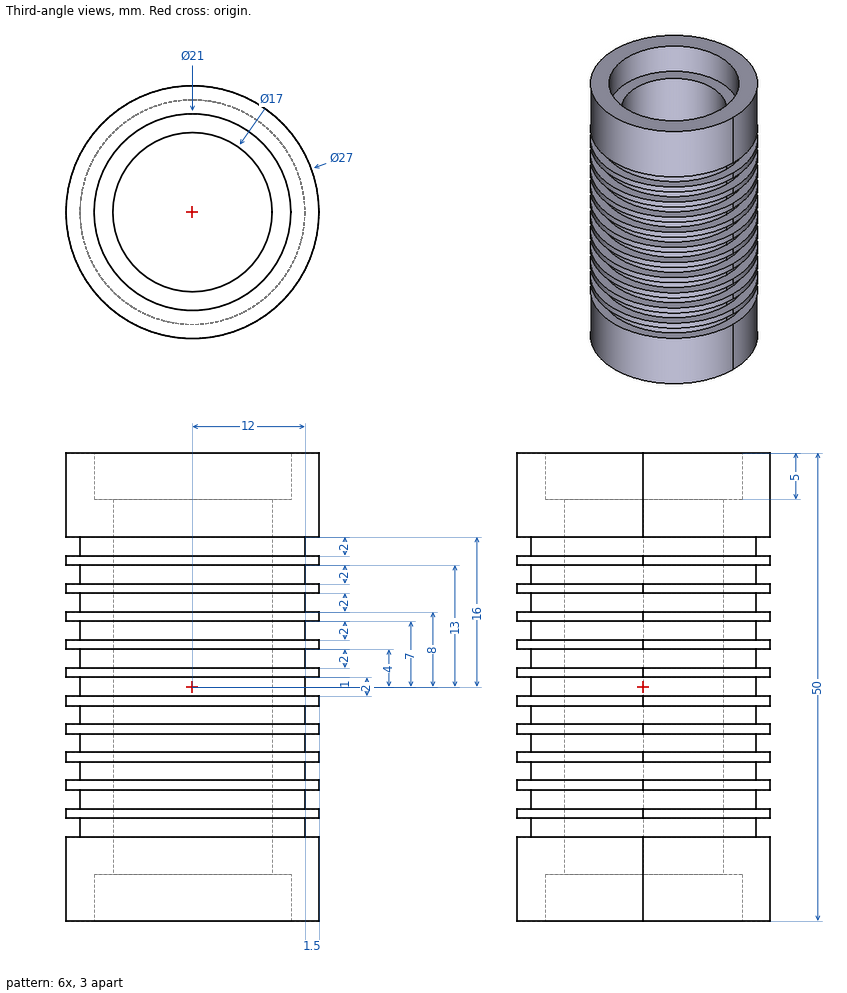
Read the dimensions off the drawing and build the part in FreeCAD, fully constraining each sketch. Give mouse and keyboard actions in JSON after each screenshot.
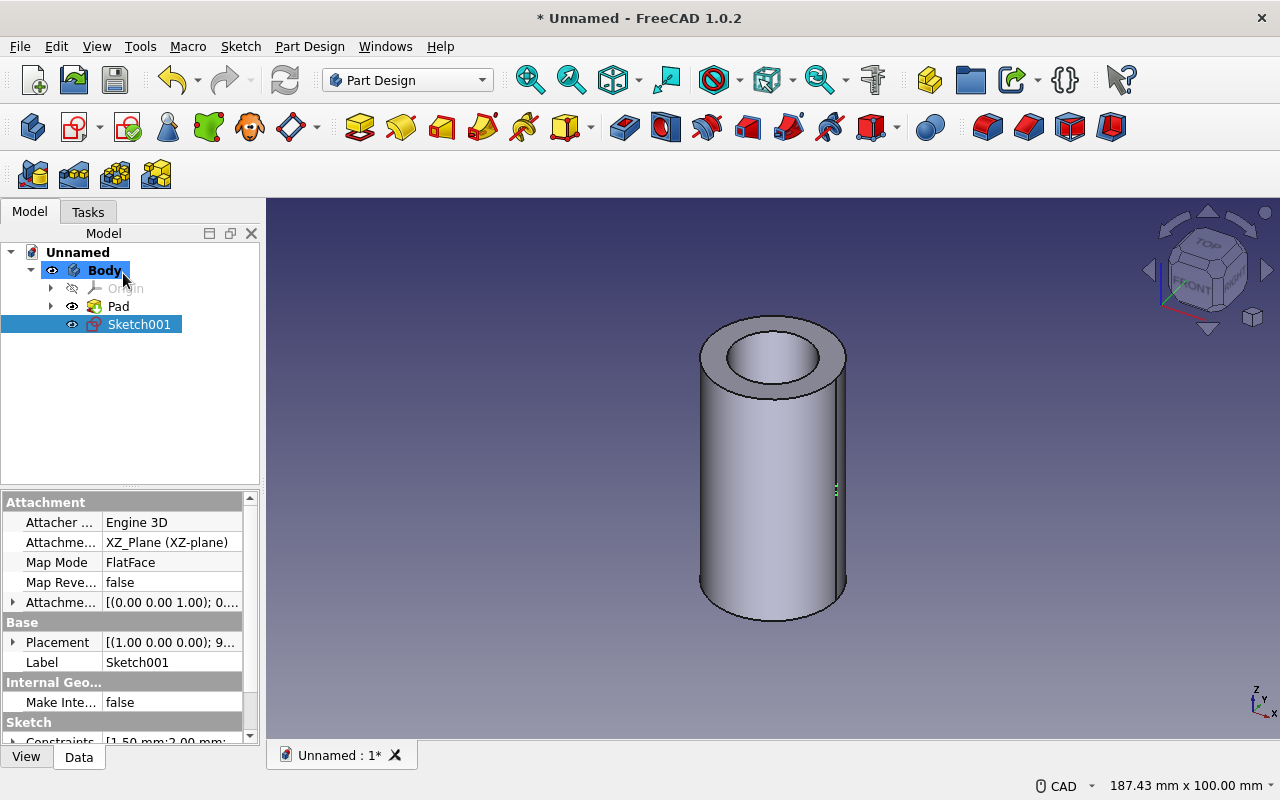
{"action": "left_click", "coordinate": [707, 128]}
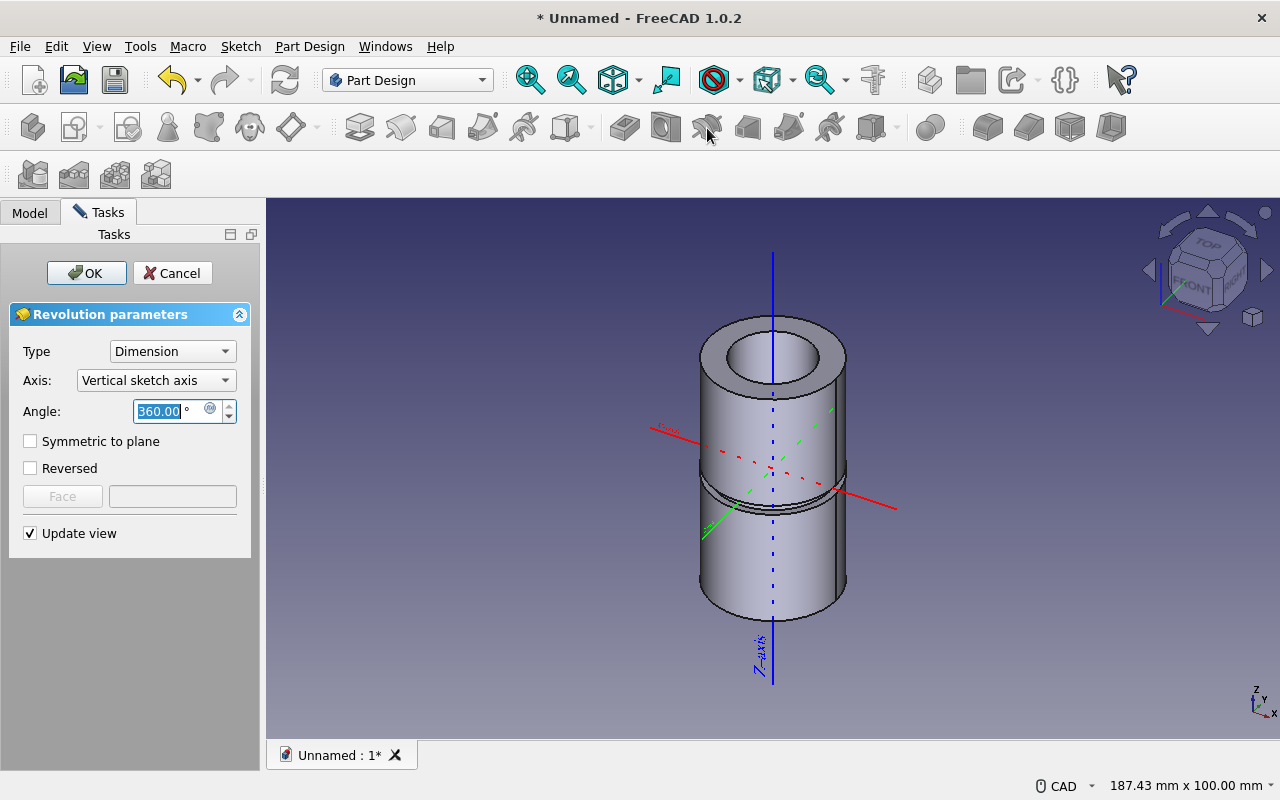
{"action": "left_click", "coordinate": [87, 273]}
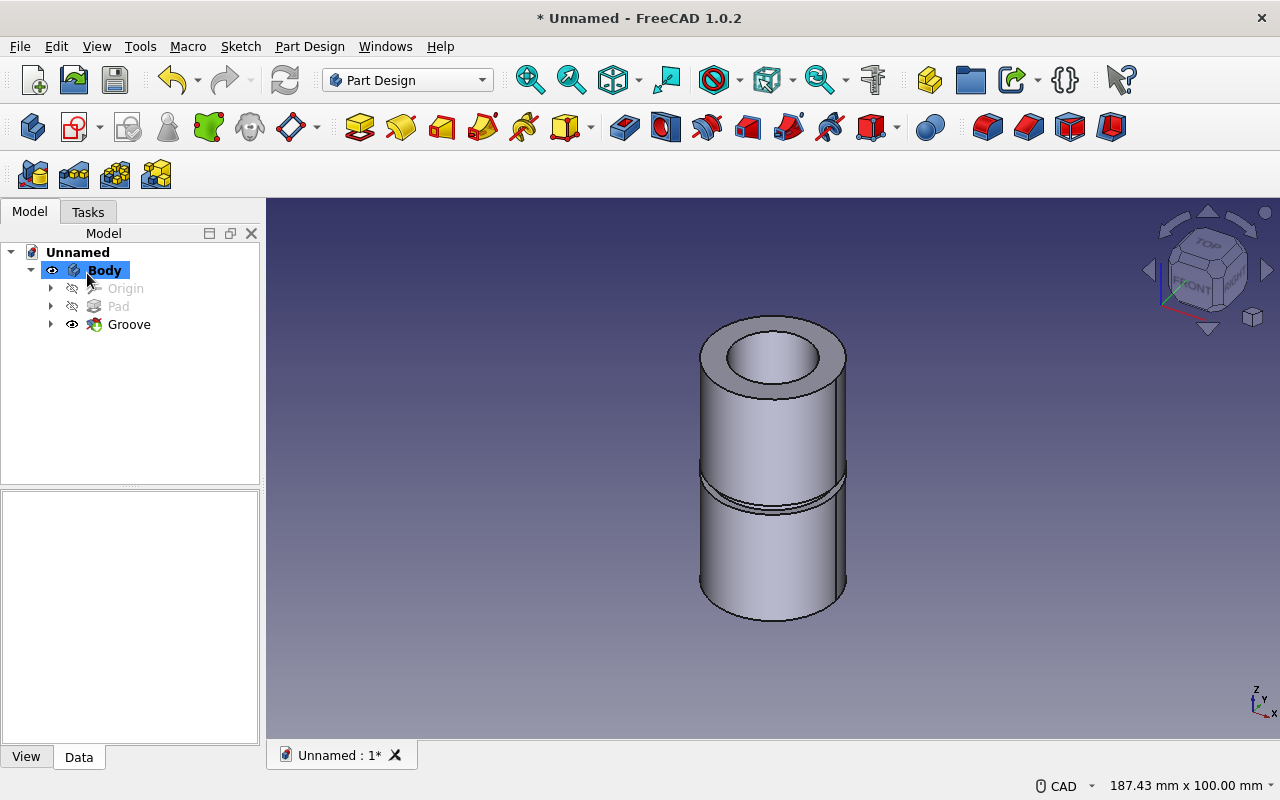
{"action": "left_click", "coordinate": [117, 324]}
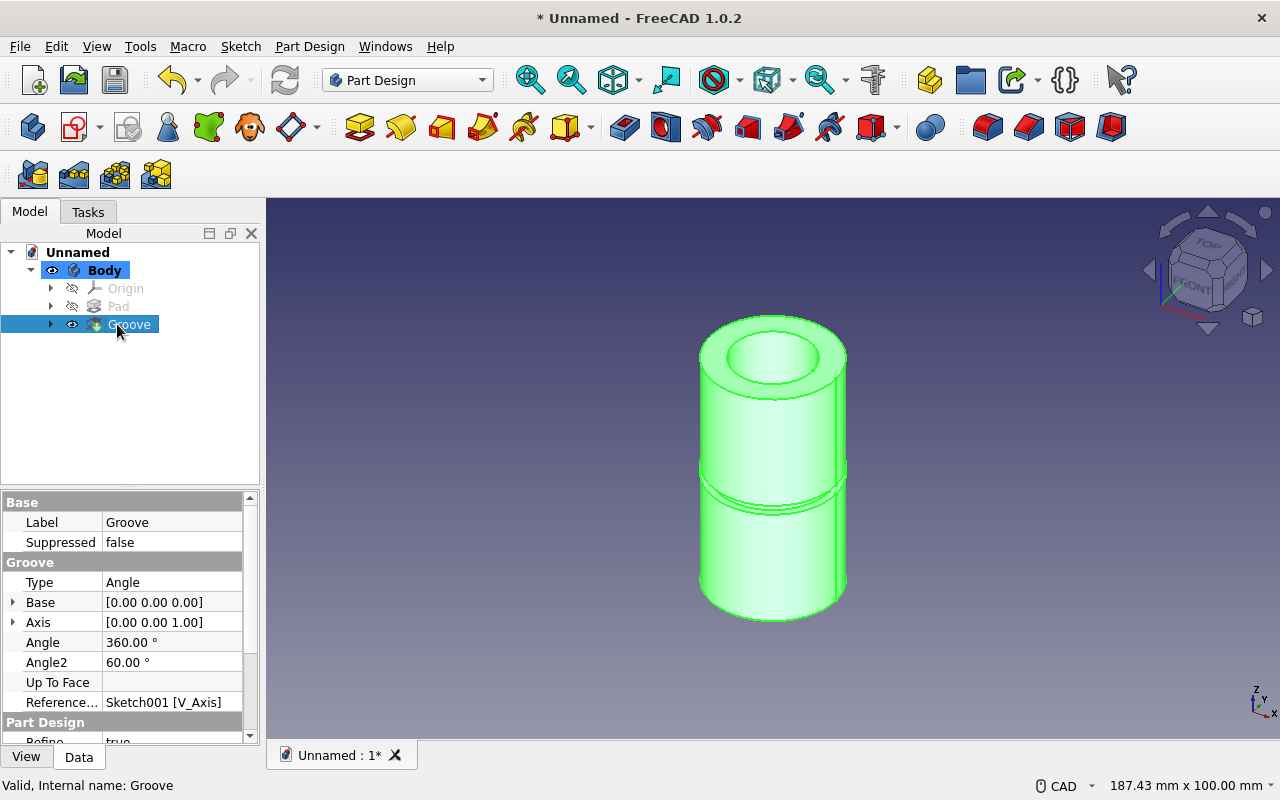
{"action": "left_click", "coordinate": [74, 174]}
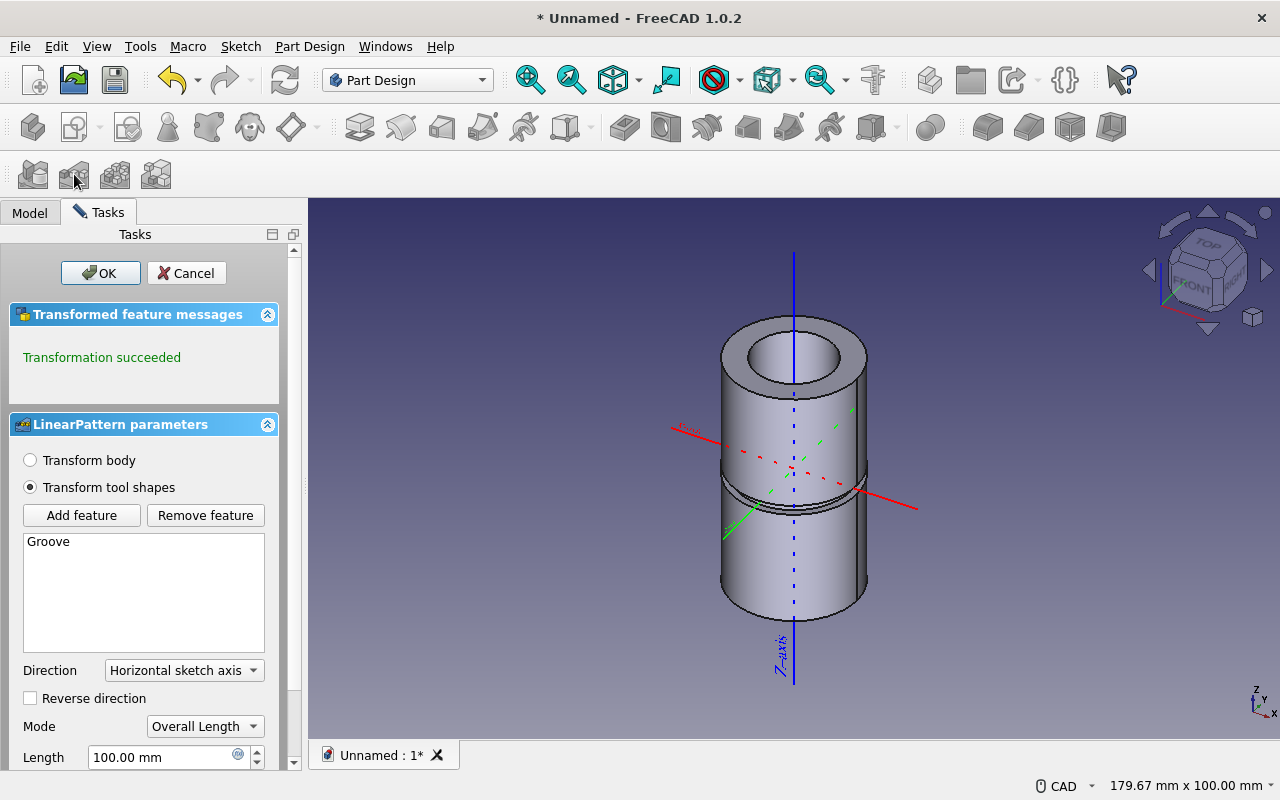
{"action": "left_click", "coordinate": [185, 670]}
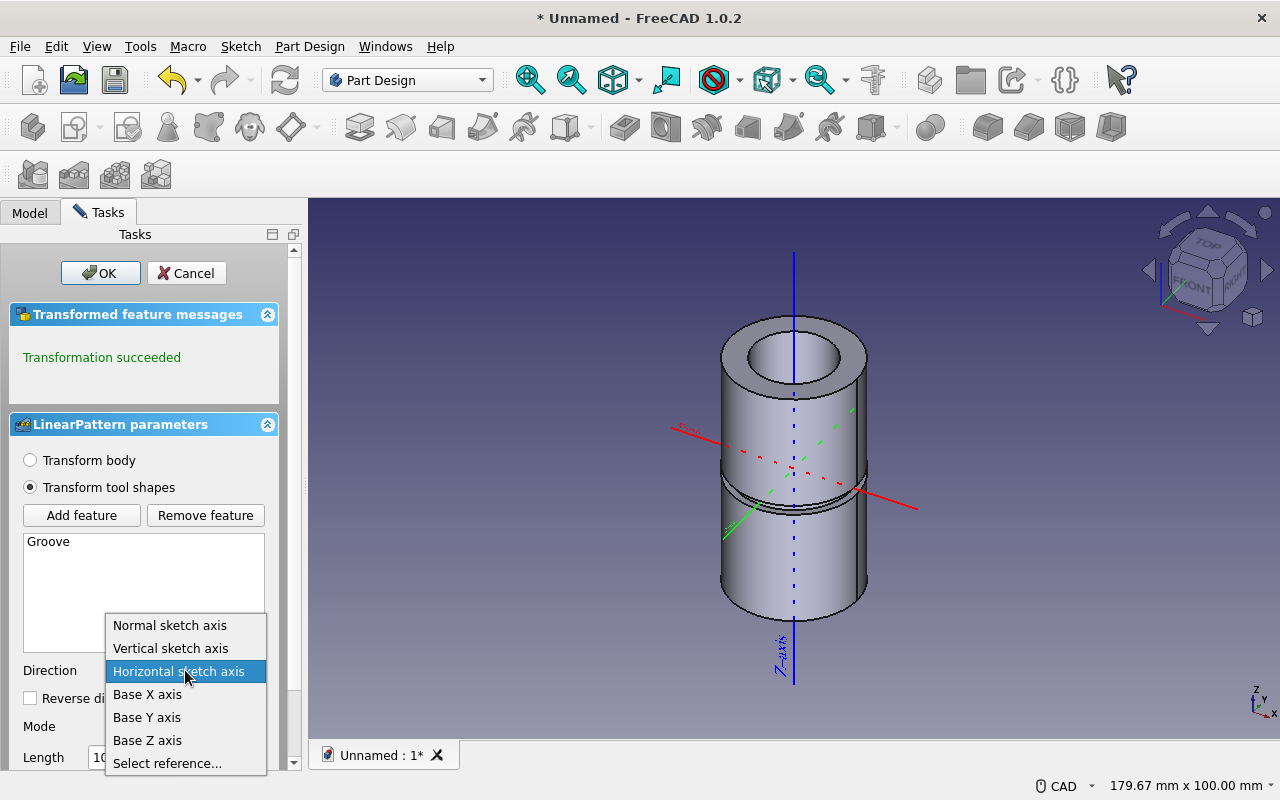
{"action": "left_click", "coordinate": [184, 740]}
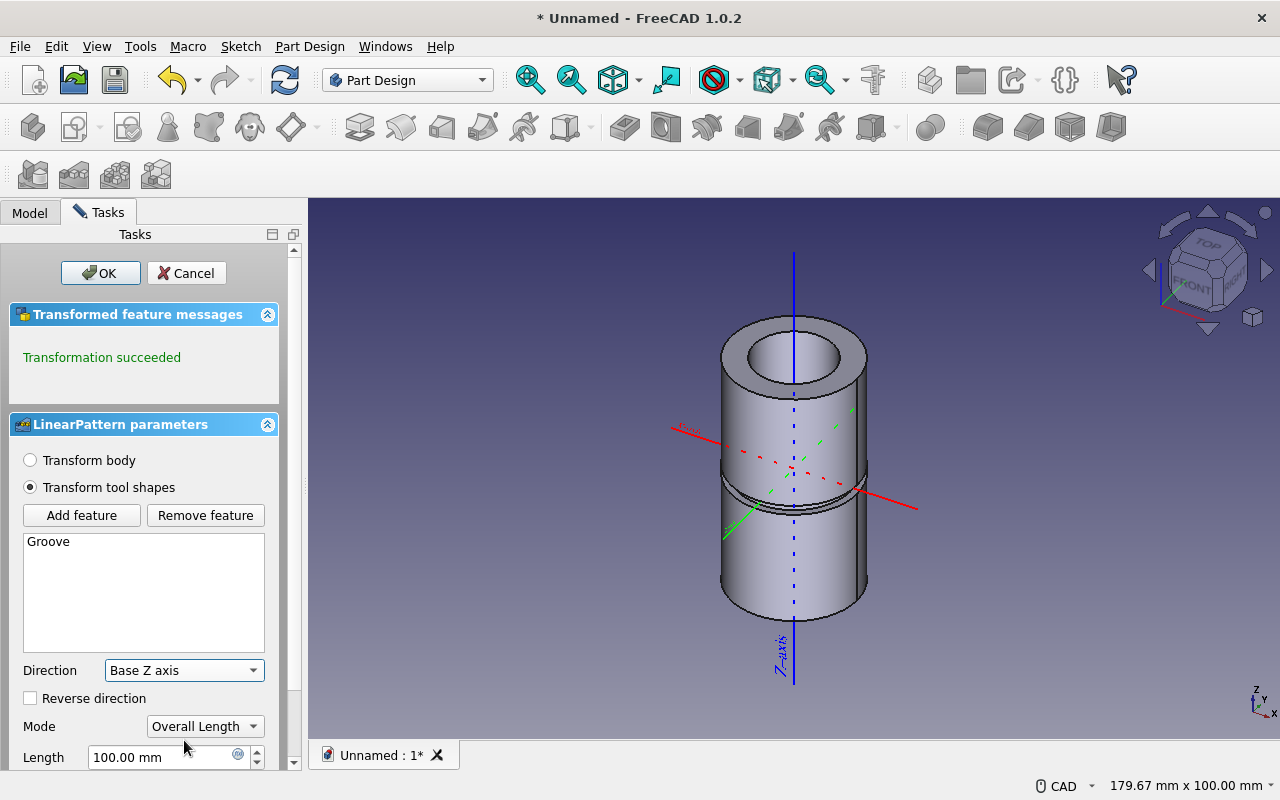
{"action": "left_click", "coordinate": [206, 726]}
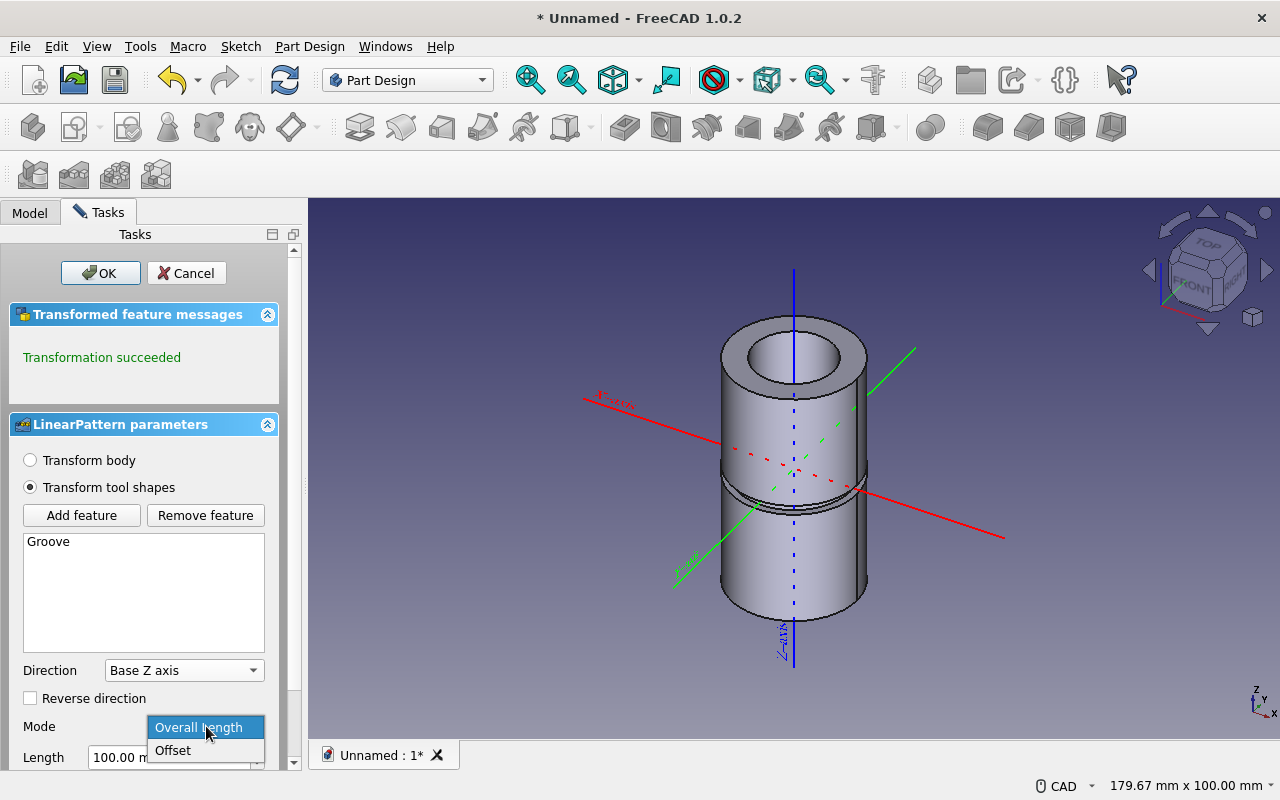
{"action": "left_click", "coordinate": [204, 750]}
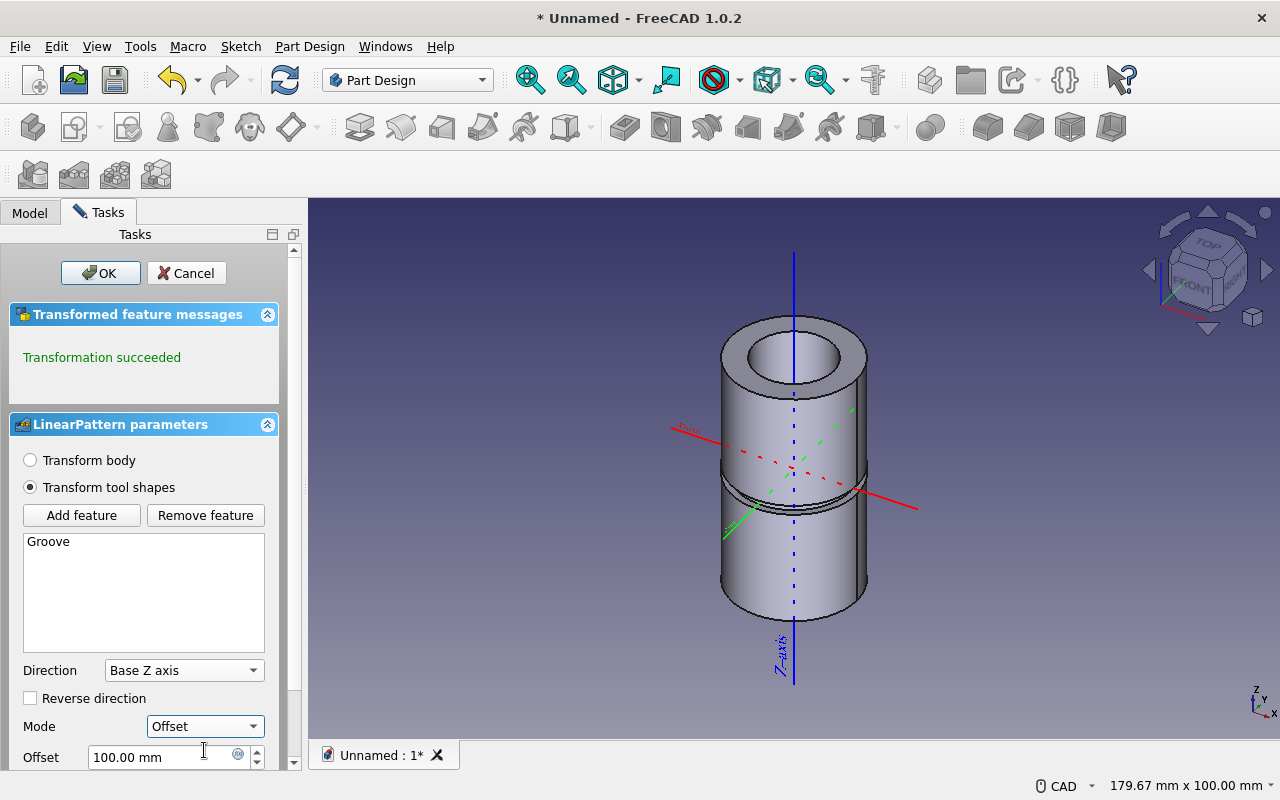
{"action": "scroll", "coordinate": [294, 507], "scroll_direction": "down", "scroll_amount": 2}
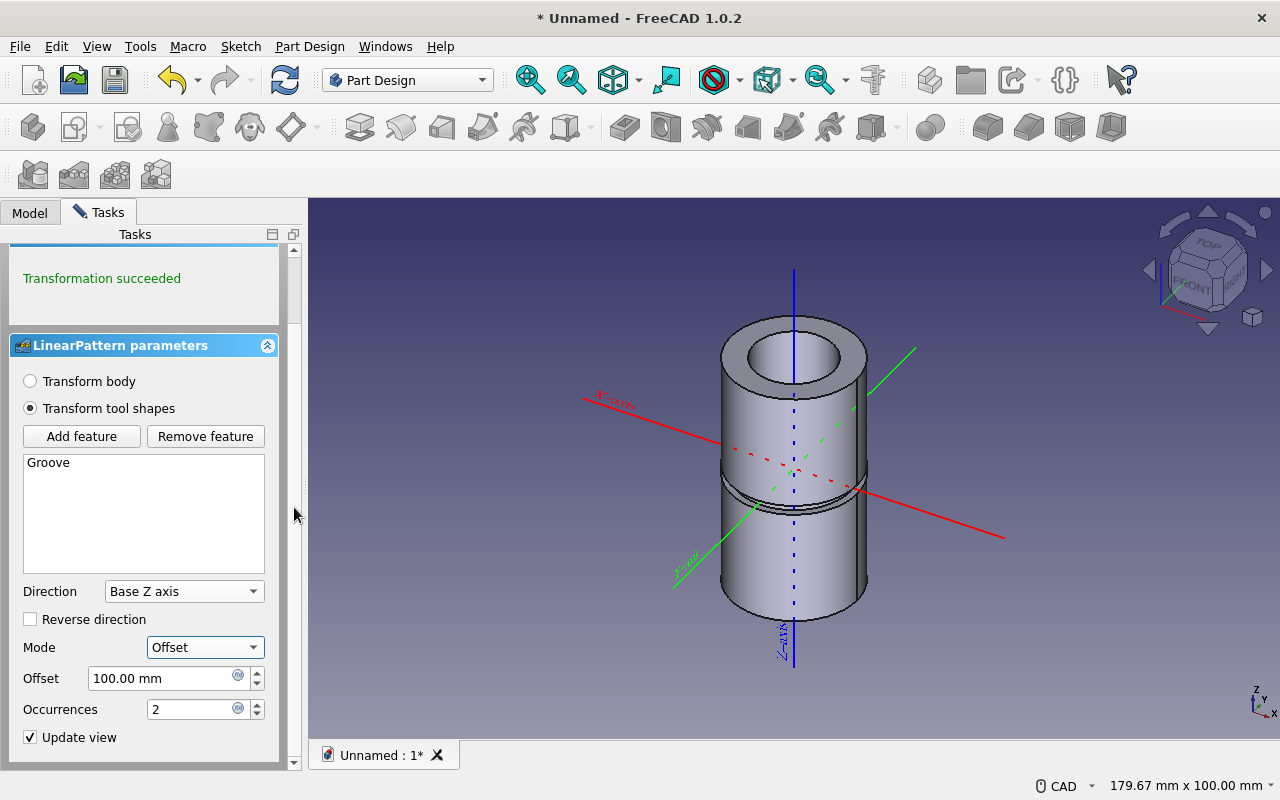
{"action": "triple_click", "coordinate": [170, 678]}